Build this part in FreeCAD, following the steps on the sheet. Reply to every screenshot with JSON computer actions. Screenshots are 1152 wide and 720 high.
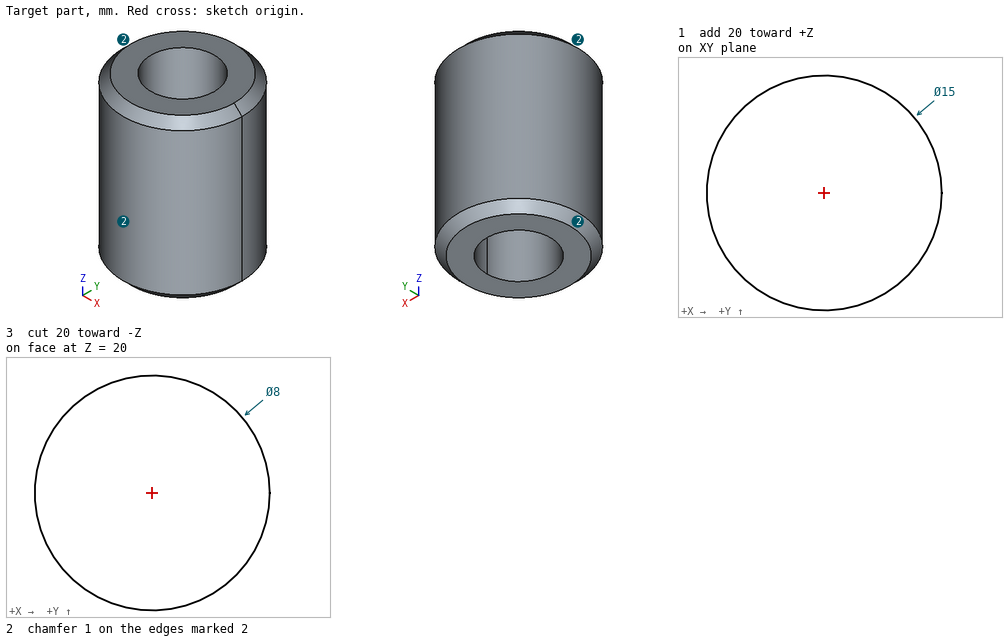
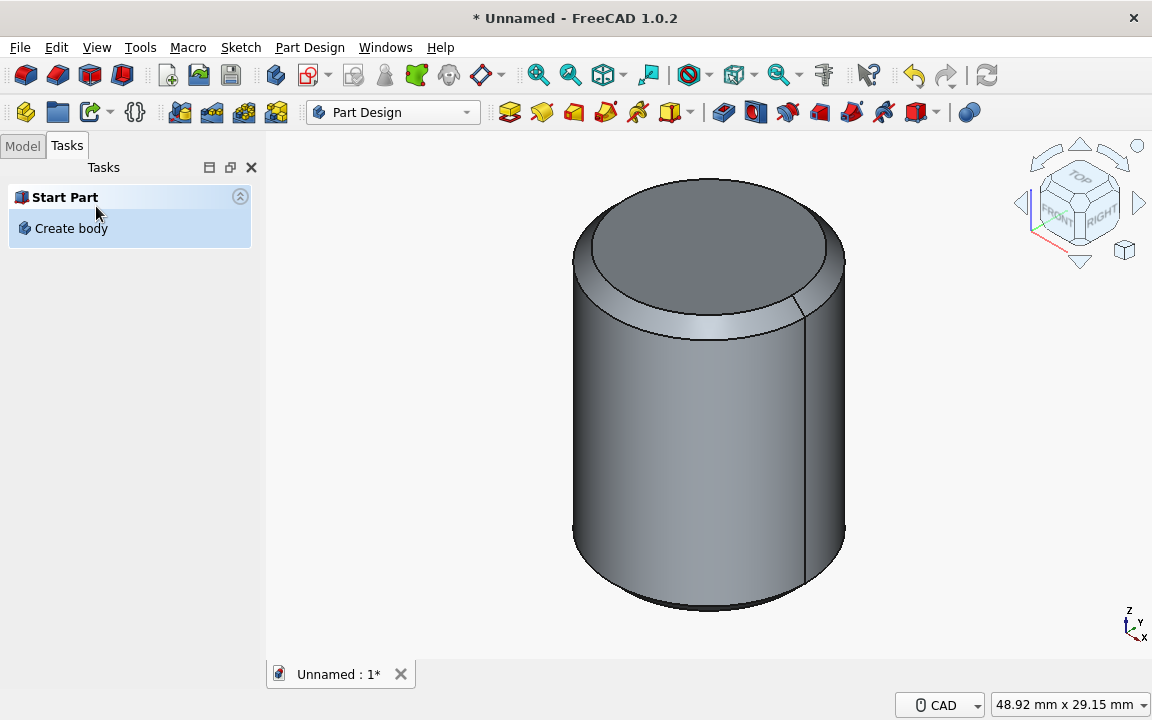
{"action": "left_click", "coordinate": [709, 246]}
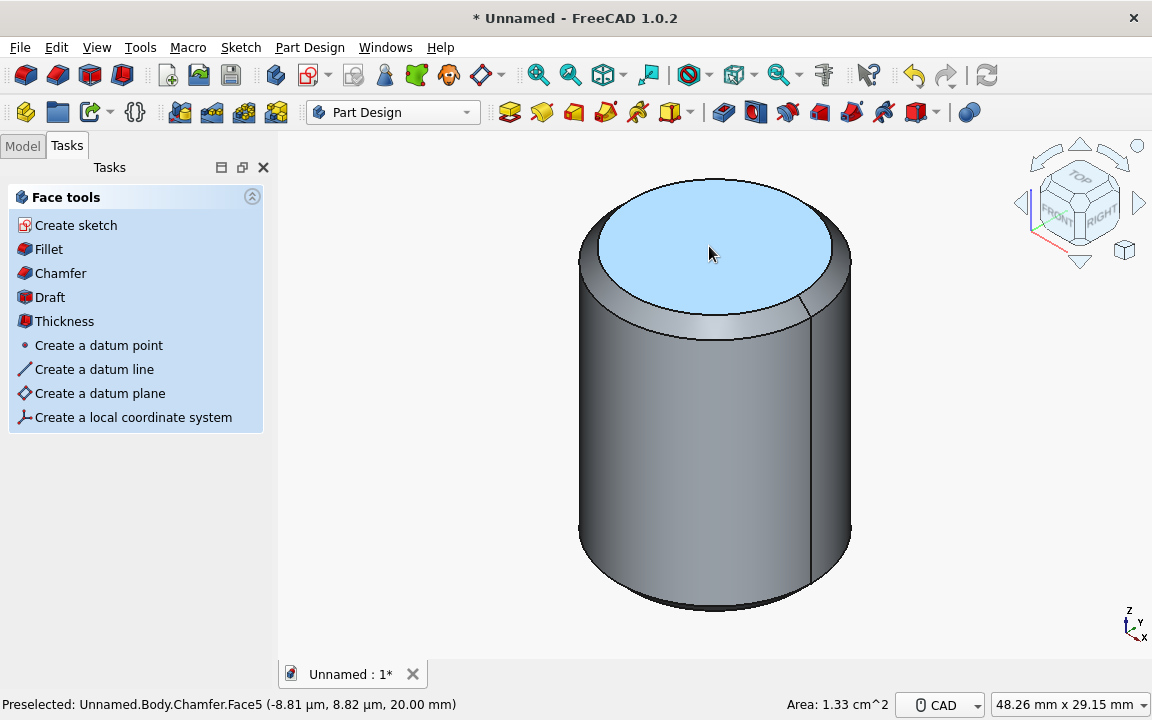
{"action": "left_click", "coordinate": [308, 76]}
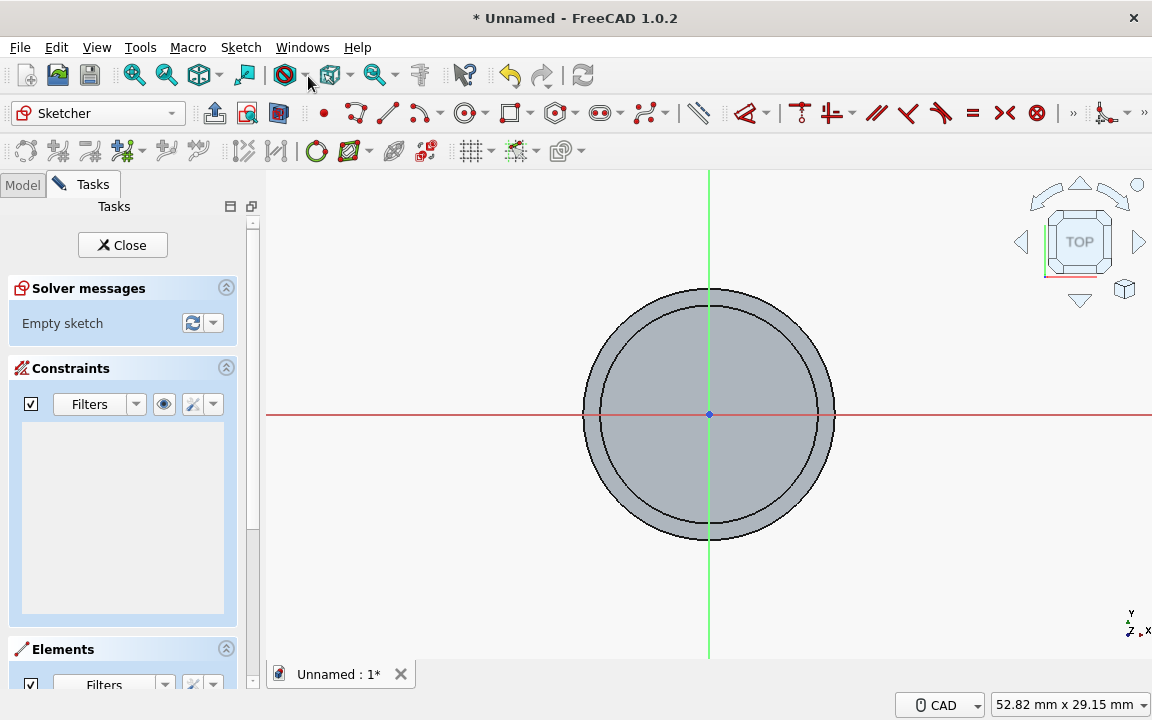
{"action": "scroll", "coordinate": [765, 415], "scroll_direction": "up", "scroll_amount": 4}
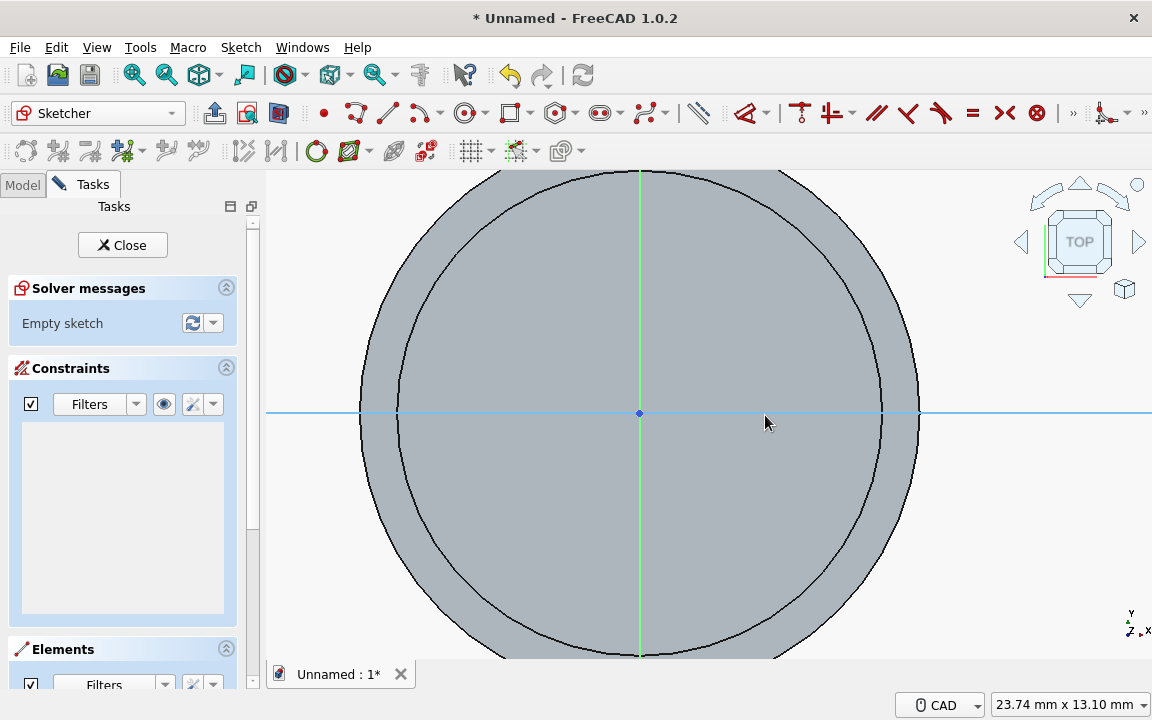
{"action": "key", "text": "g c"}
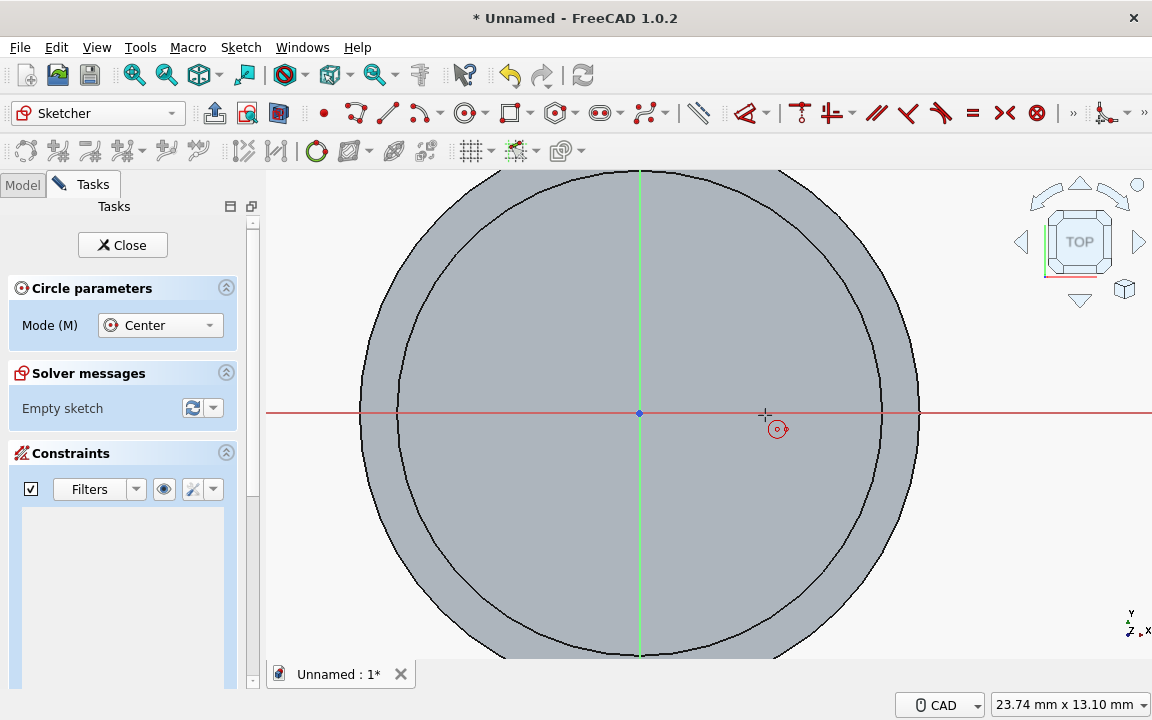
{"action": "left_click", "coordinate": [640, 413]}
{"action": "left_click", "coordinate": [745, 308]}
{"action": "key", "text": "Escape"}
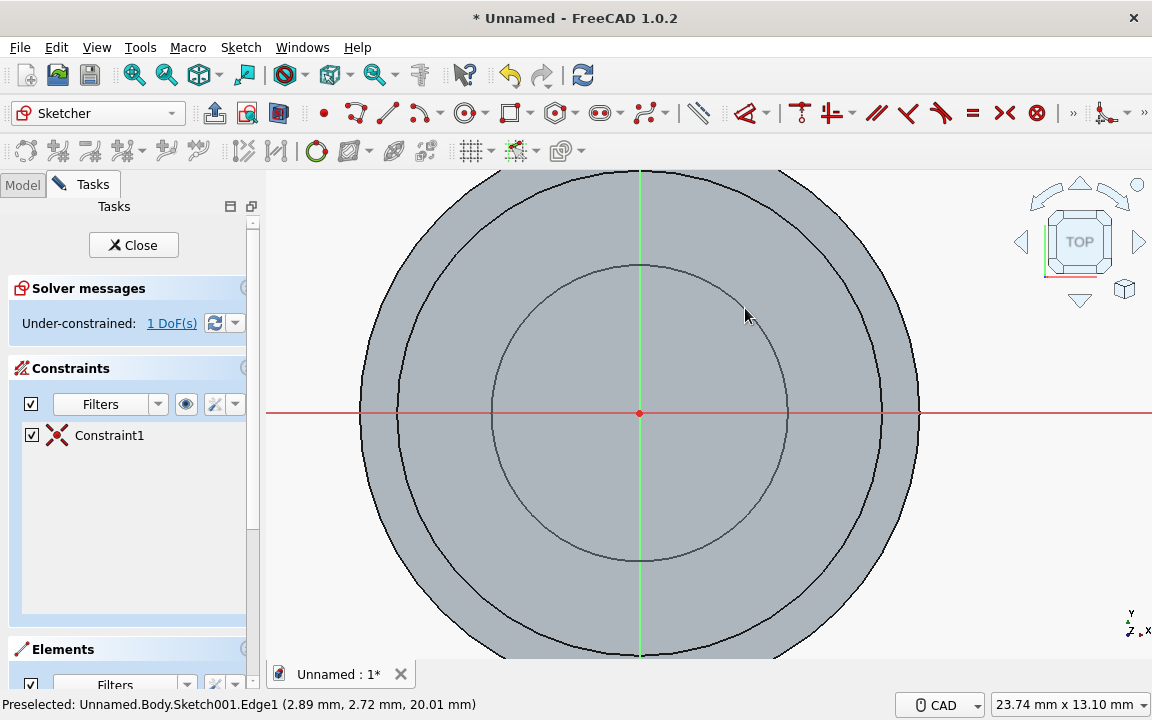
{"action": "left_click", "coordinate": [746, 114]}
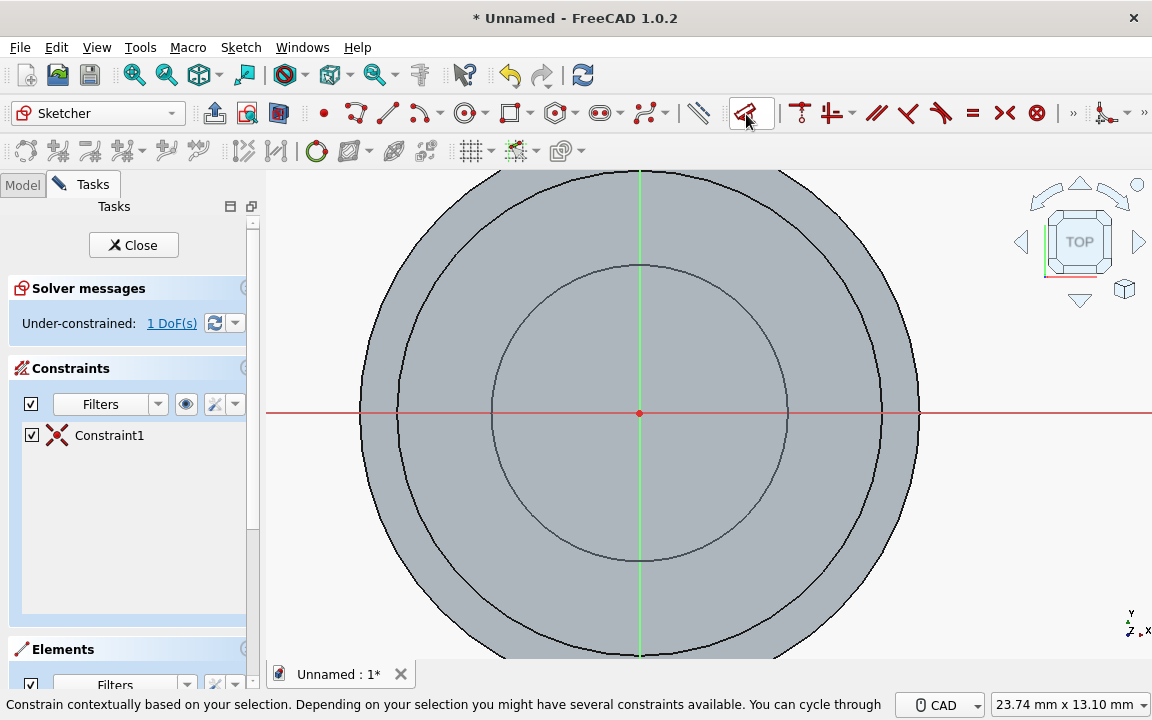
{"action": "left_click", "coordinate": [744, 308]}
{"action": "left_click", "coordinate": [767, 285]}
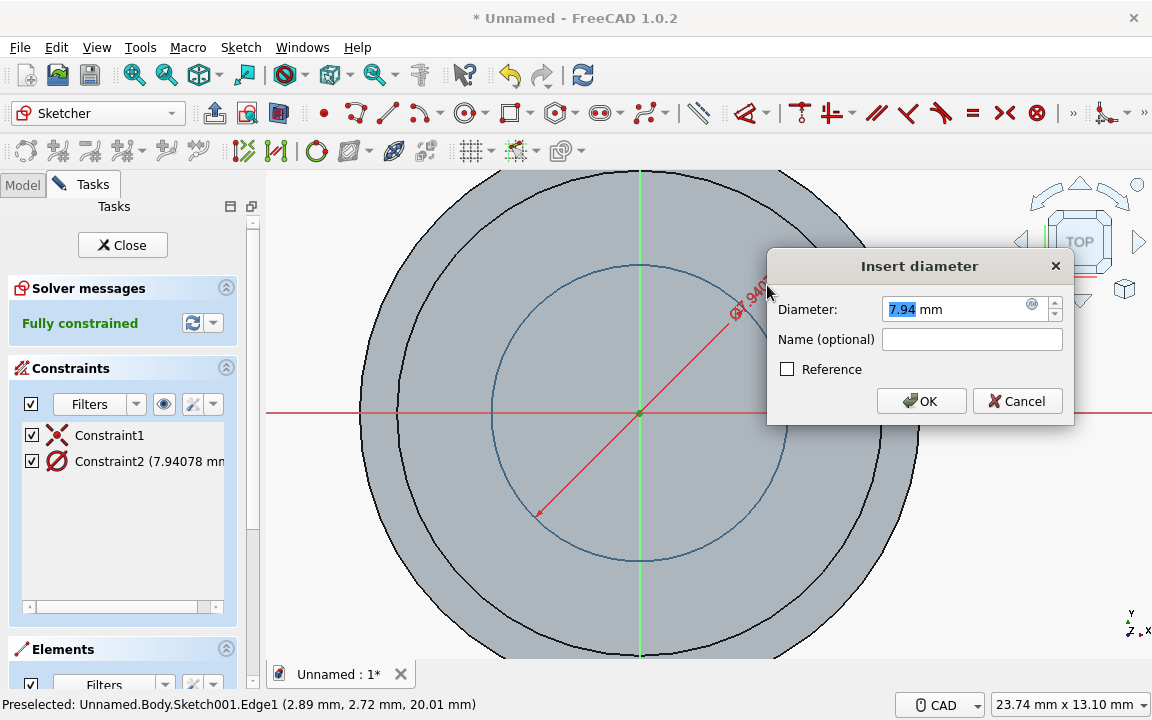
{"action": "type", "text": "8"}
{"action": "key", "text": "Return"}
{"action": "key", "text": "Escape"}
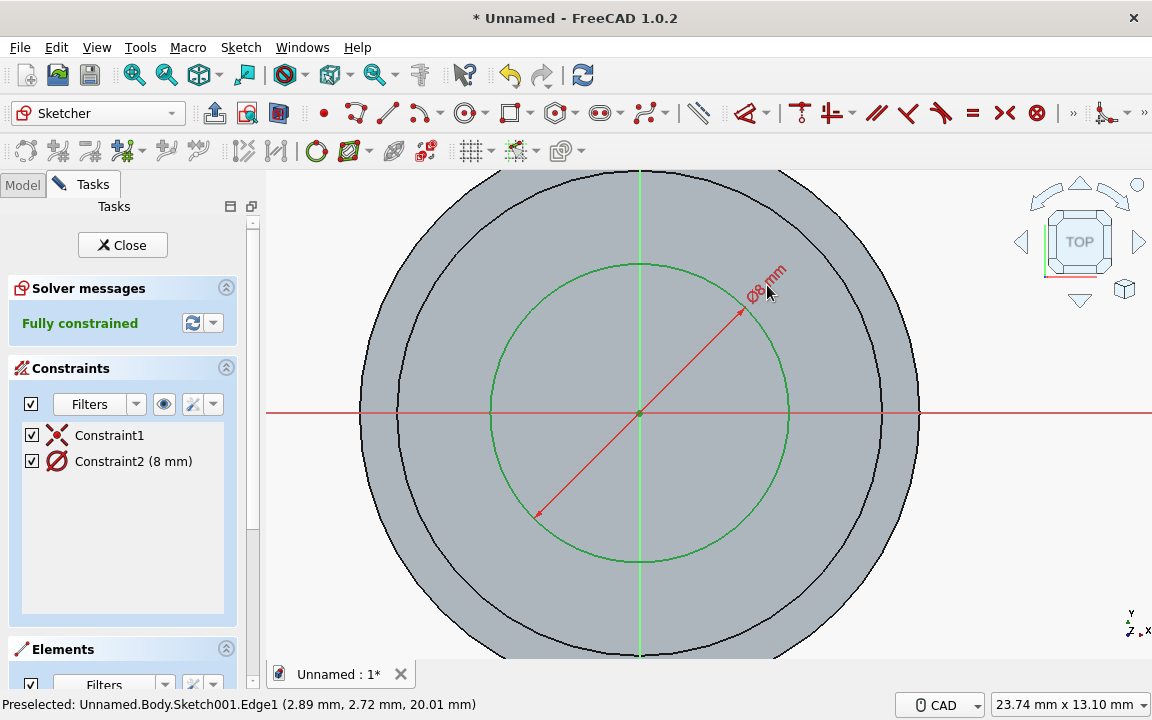
{"action": "left_click", "coordinate": [123, 245]}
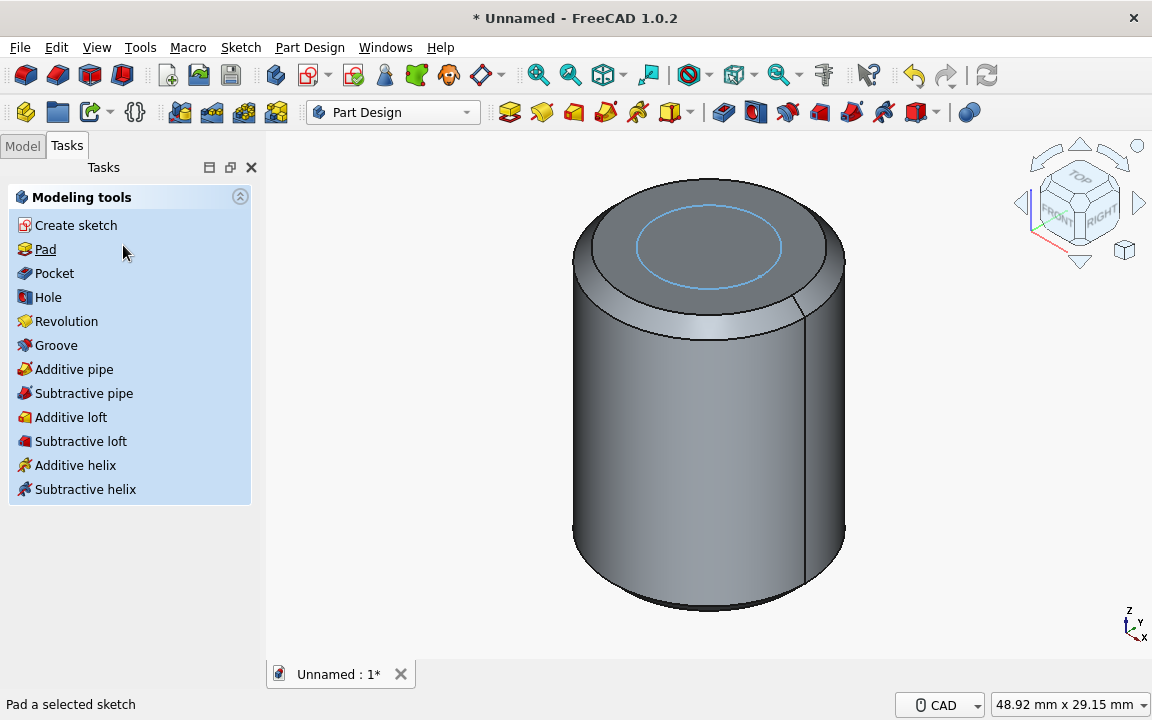
{"action": "left_click", "coordinate": [724, 112]}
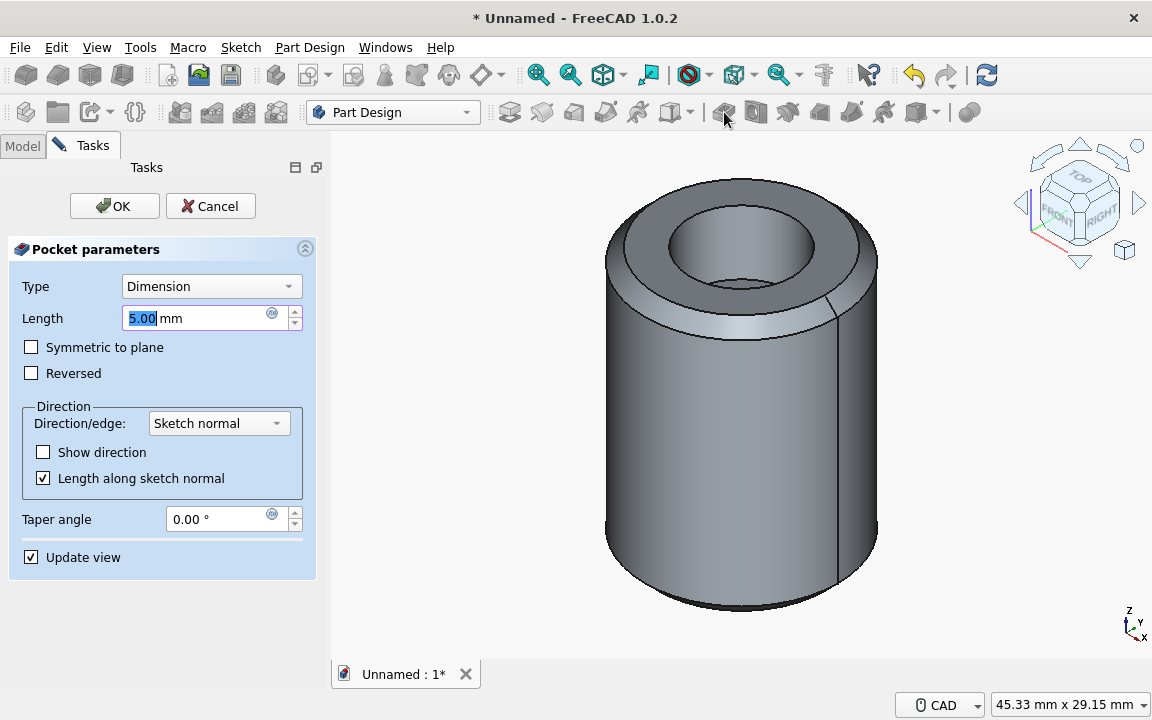
{"action": "type", "text": "20"}
{"action": "key", "text": "Tab"}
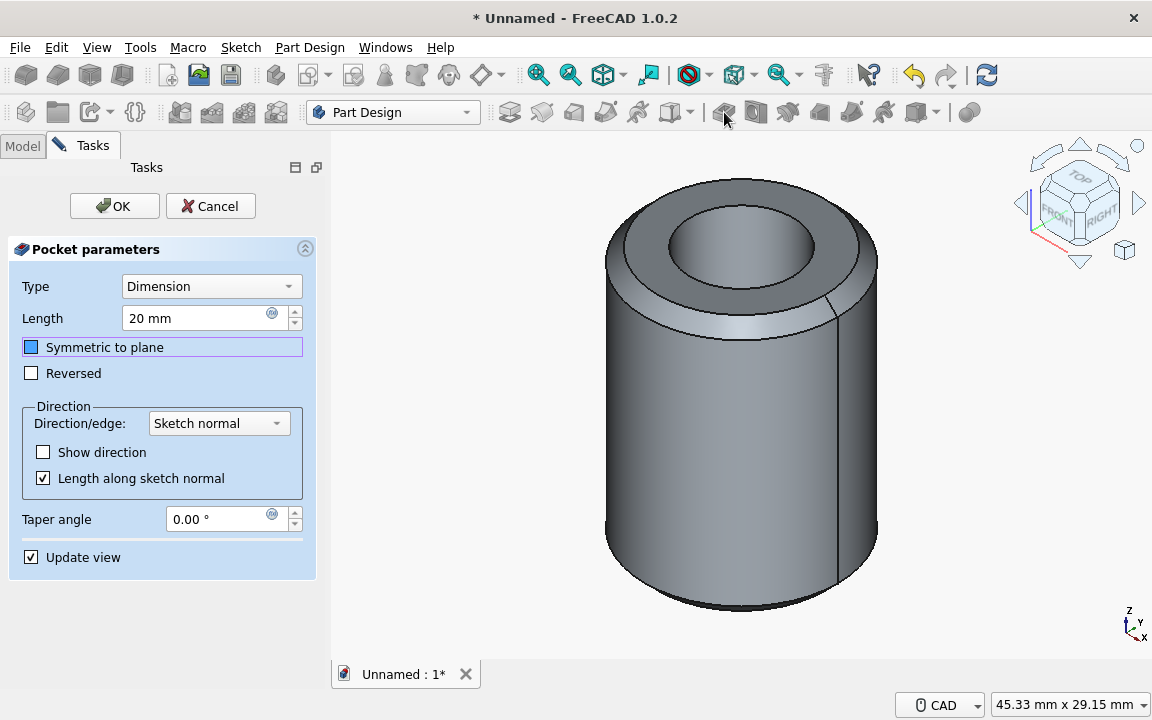
{"action": "left_click", "coordinate": [115, 206]}